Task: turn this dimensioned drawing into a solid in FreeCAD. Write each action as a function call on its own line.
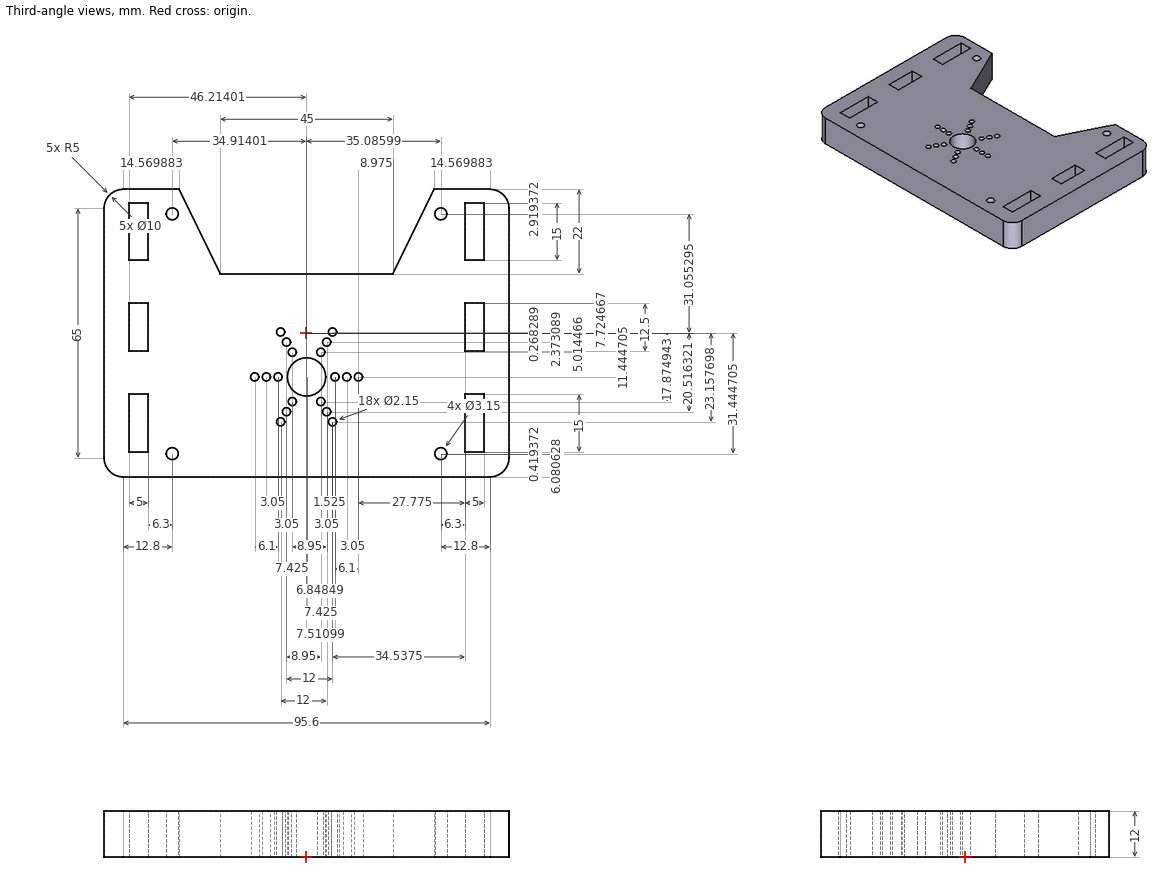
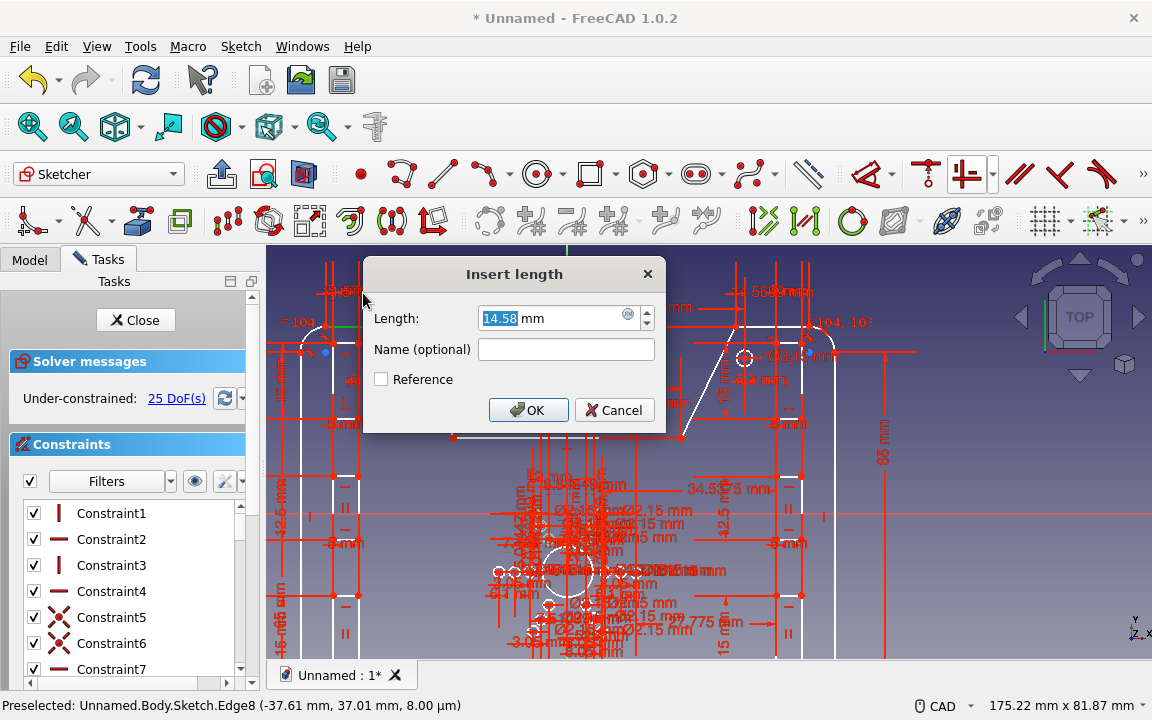
text(14.569883)
key(Return)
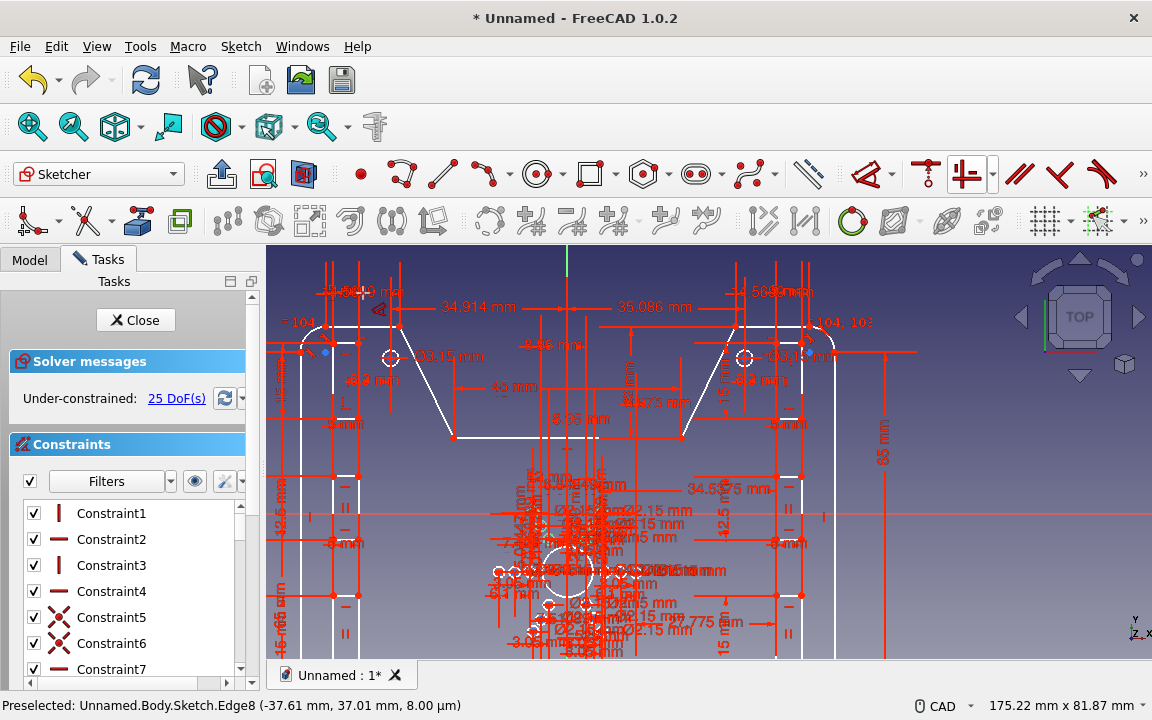
click(776, 477)
click(858, 495)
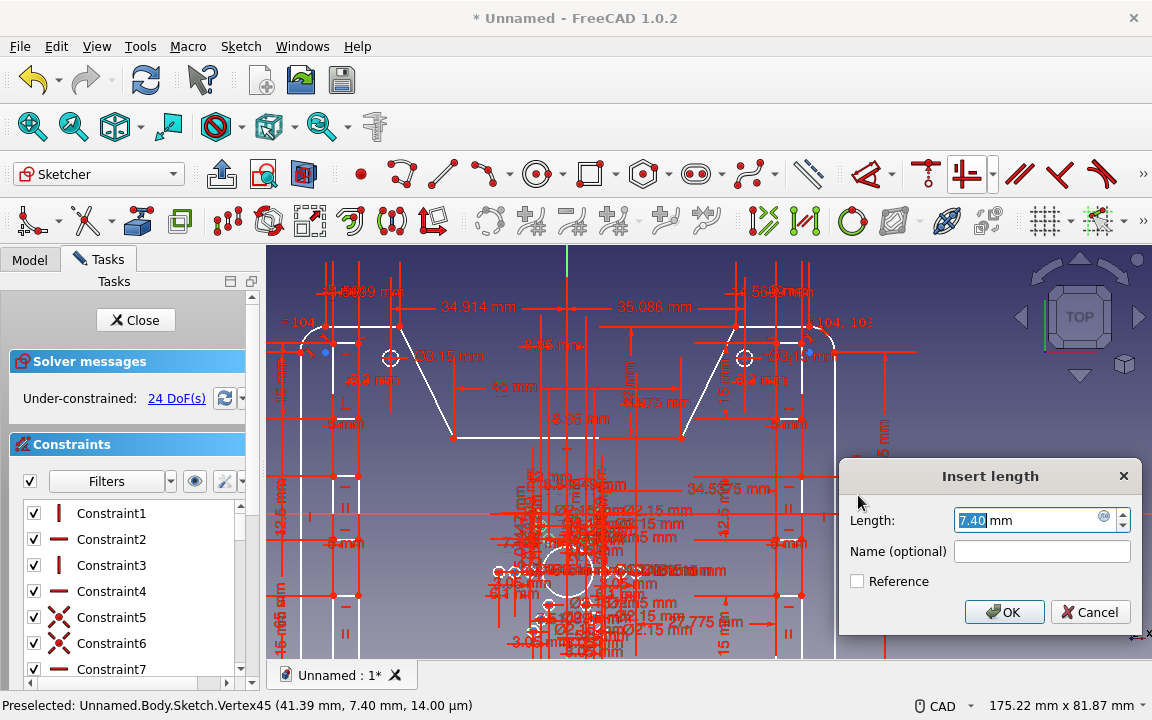
text(7.724667)
key(Return)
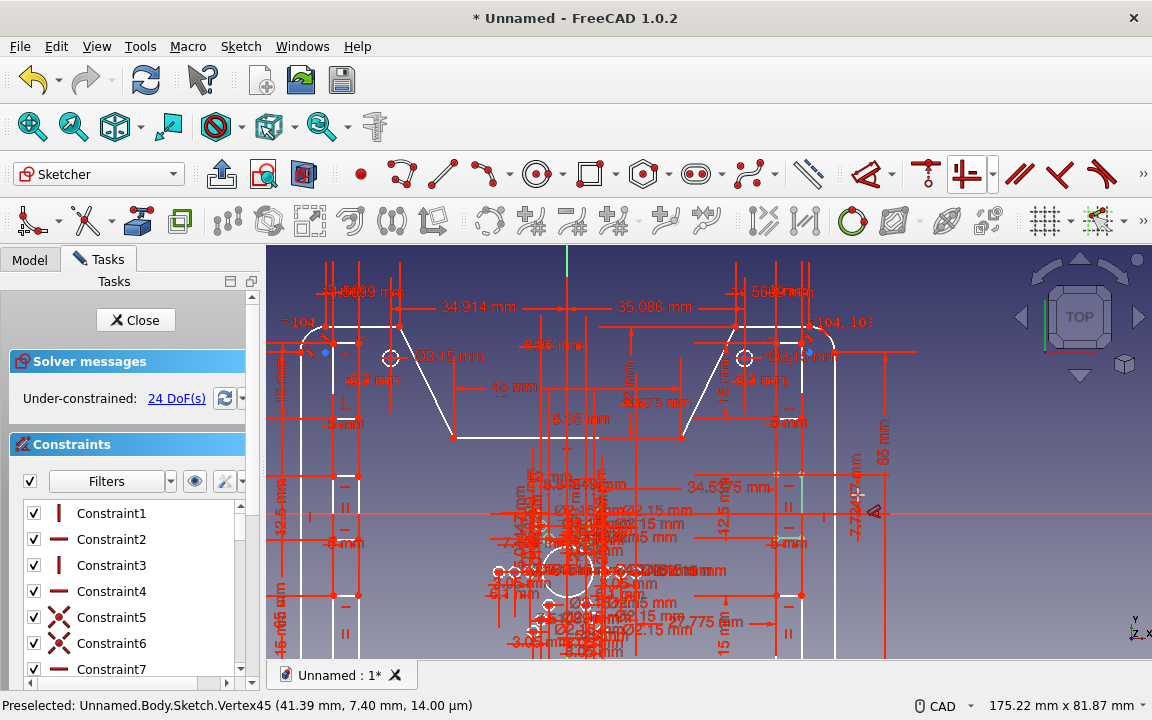
click(333, 476)
click(396, 442)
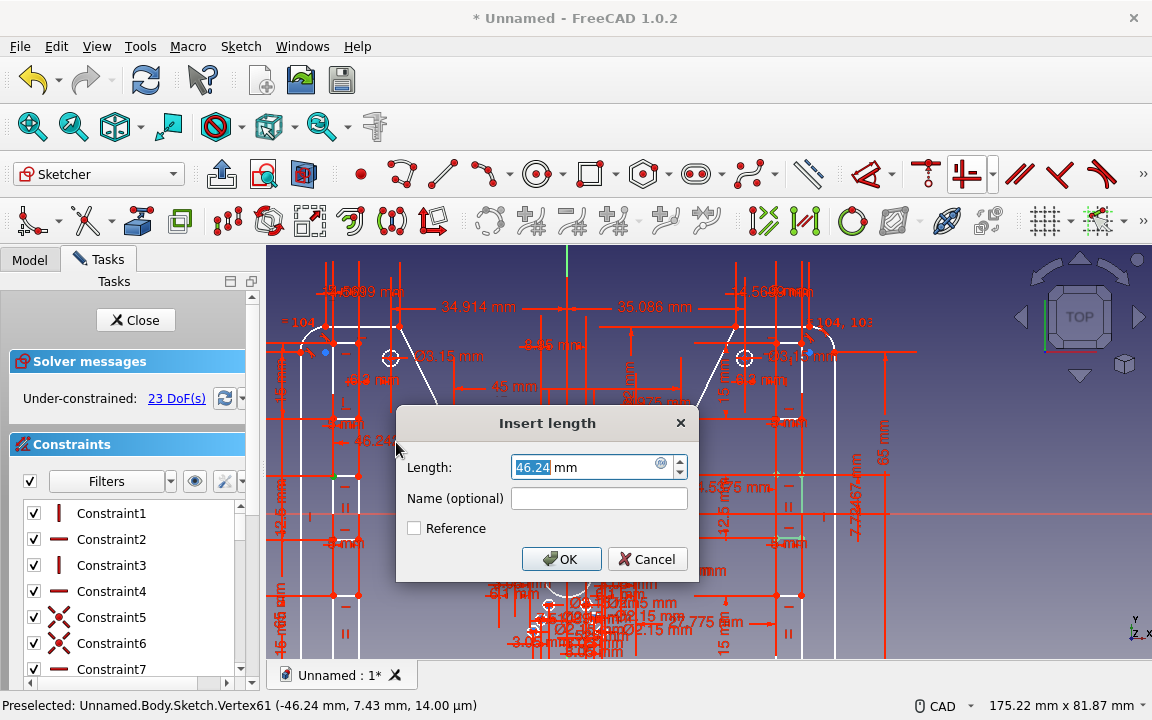
text(46.21401)
key(Return)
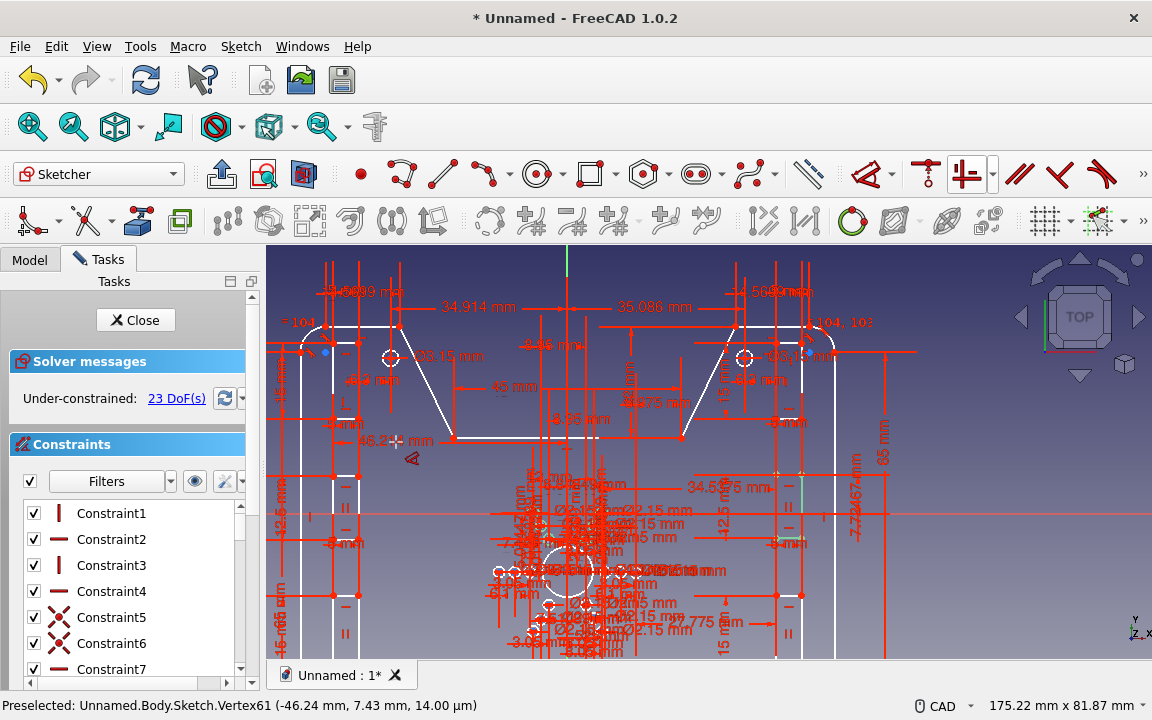
click(333, 476)
click(625, 495)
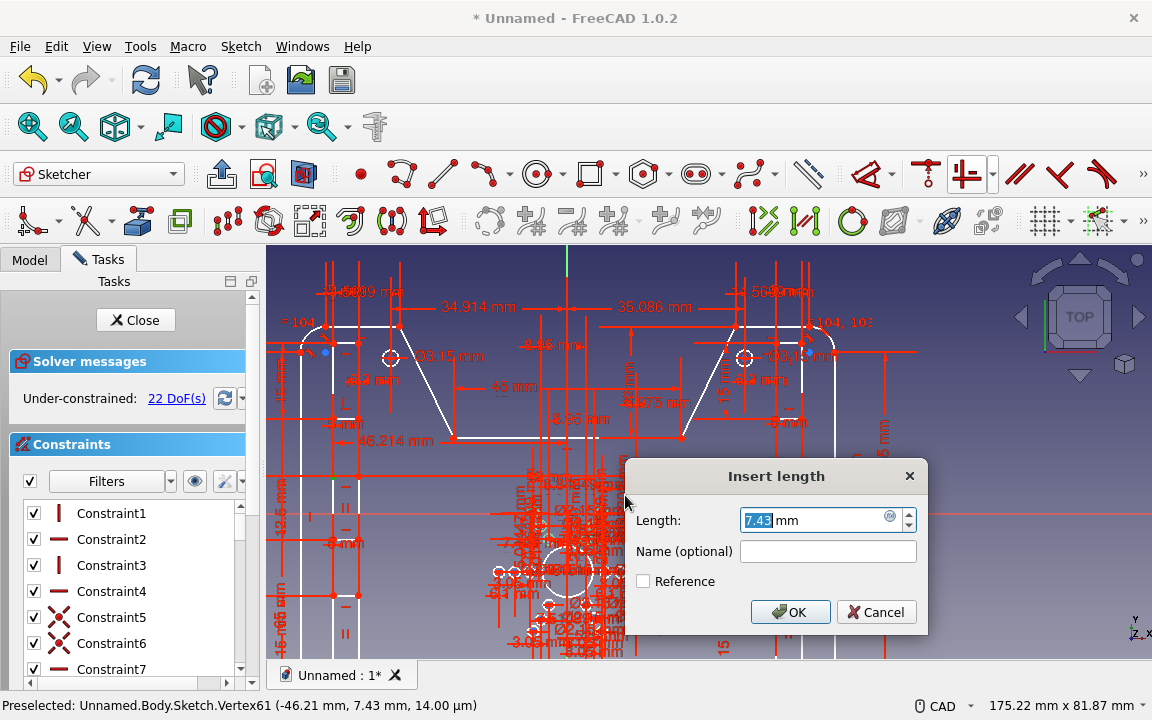
text(7.724667)
key(Return)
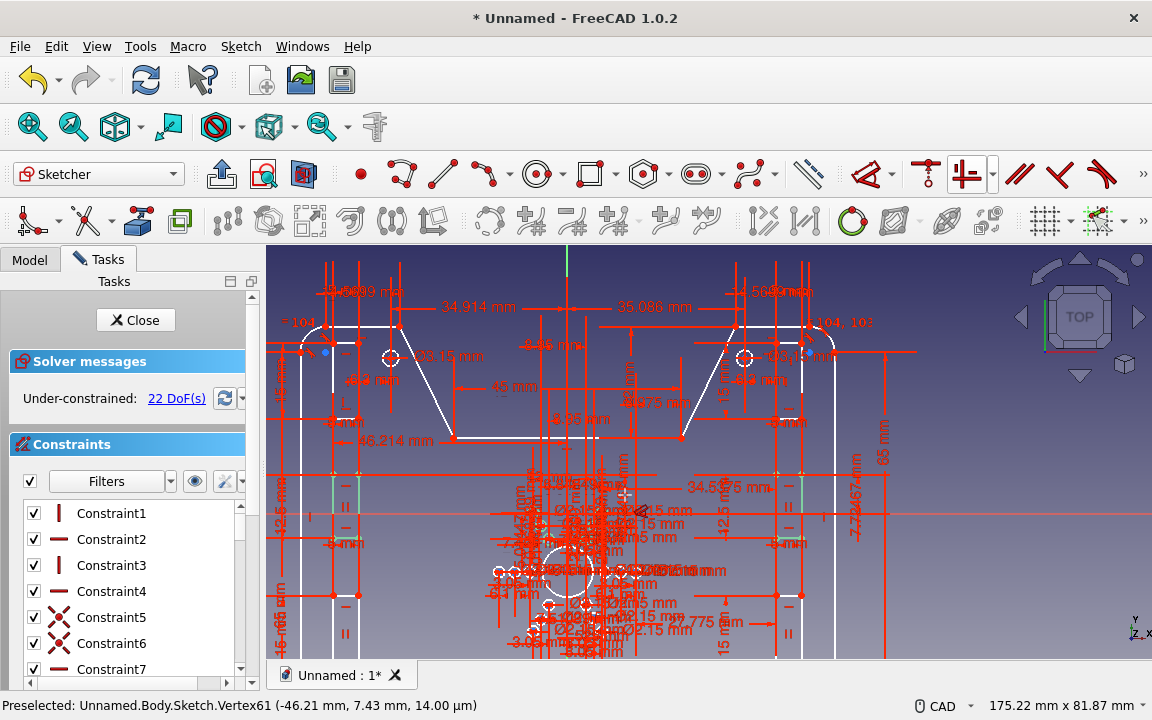
scroll(789, 326, down, 2)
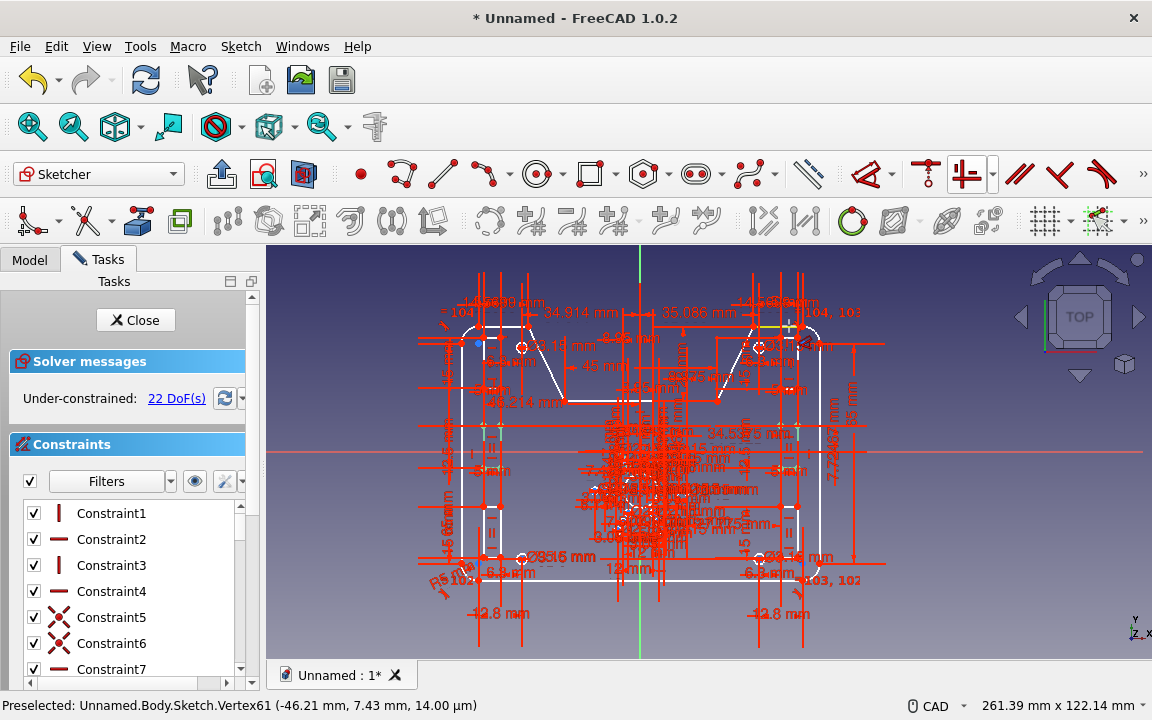
click(759, 559)
click(841, 506)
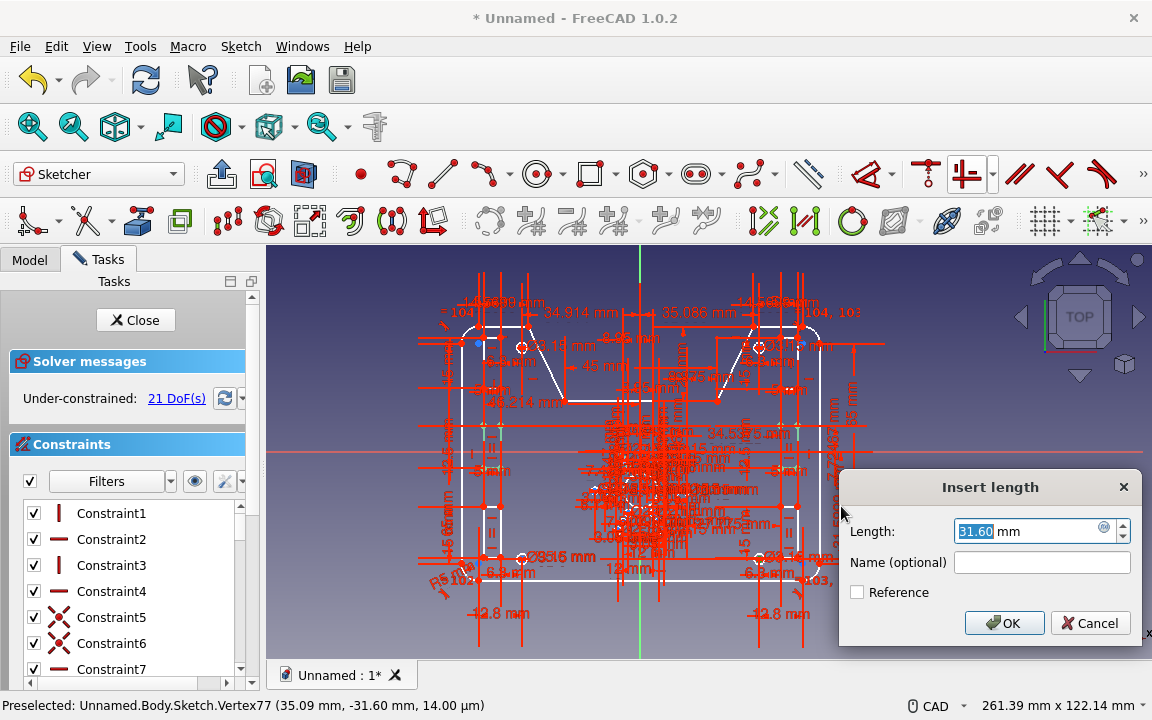
text(31.444705)
key(Return)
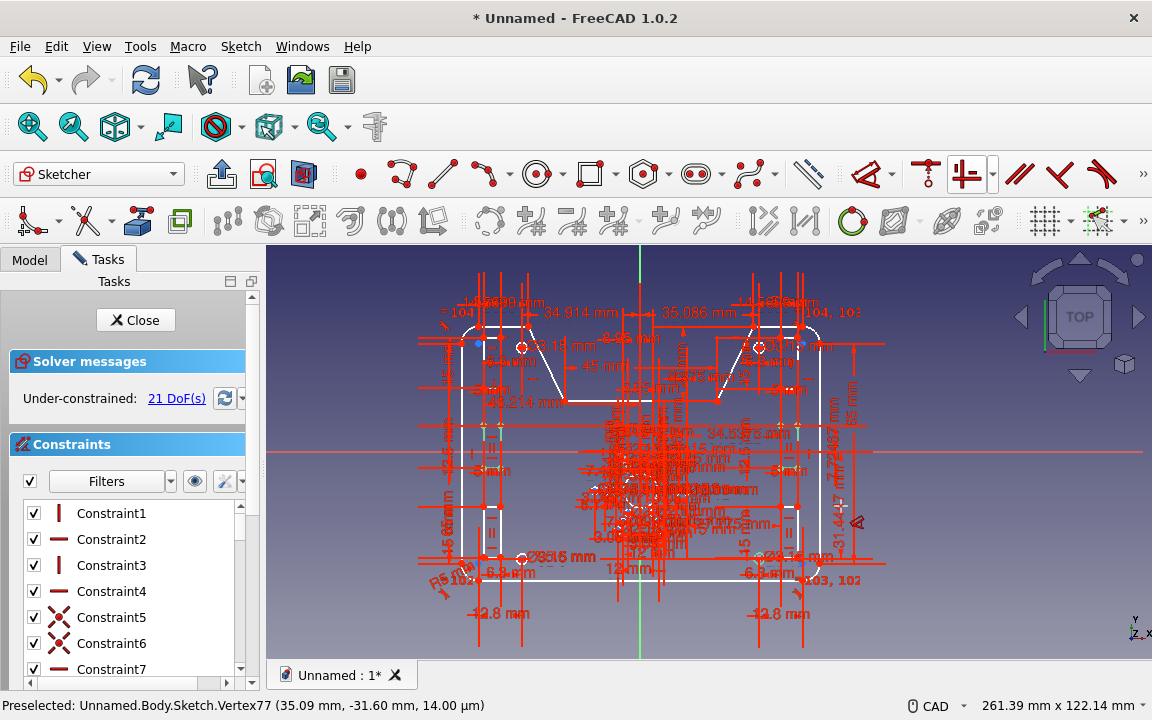
click(664, 531)
click(746, 473)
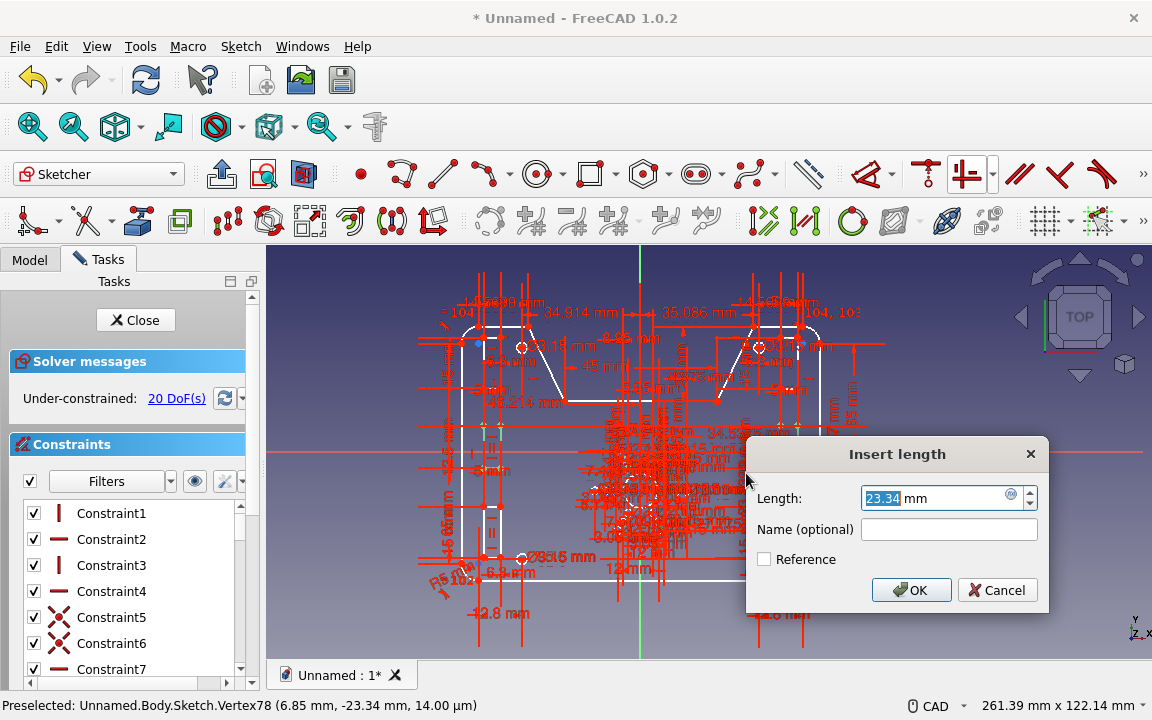
text(23.157698)
key(Return)